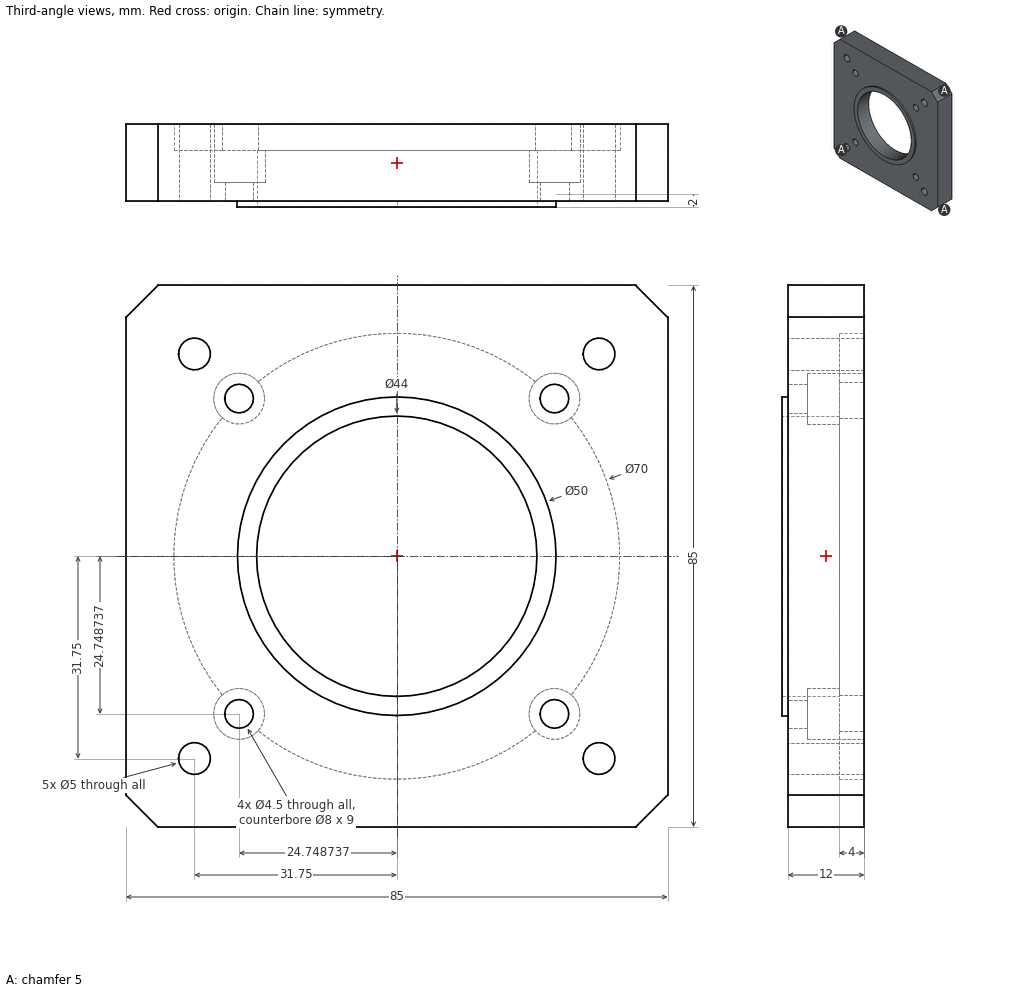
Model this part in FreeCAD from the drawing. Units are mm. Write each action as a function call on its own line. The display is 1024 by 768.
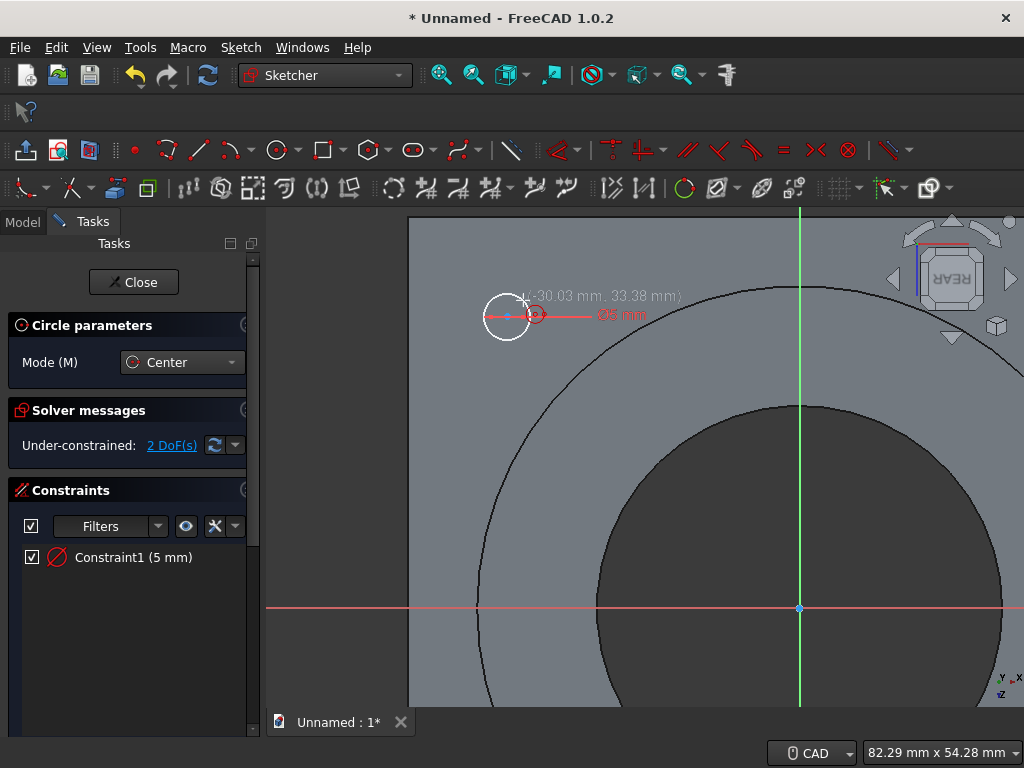
click(800, 608)
move(816, 592)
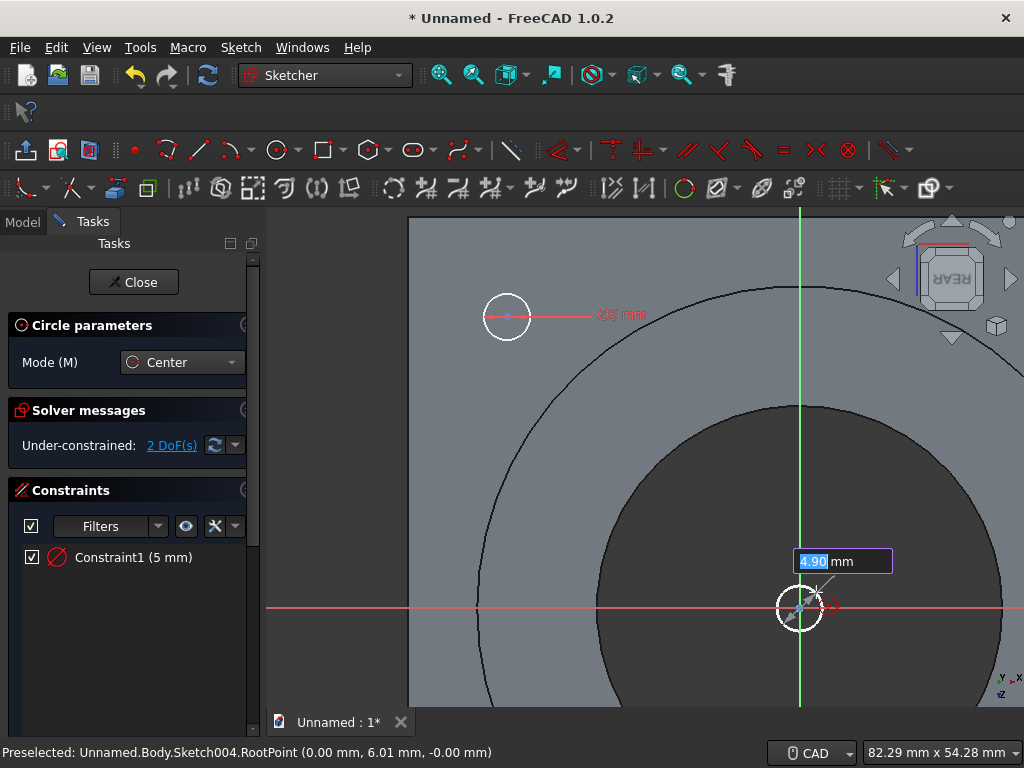
text(5)
key(Return)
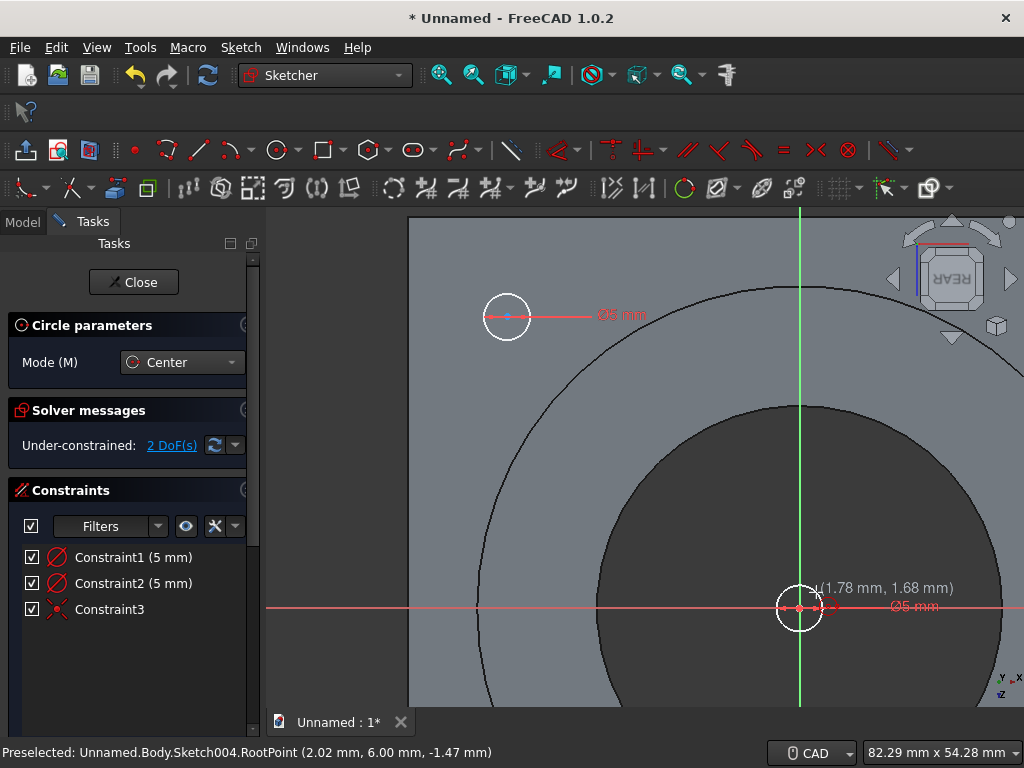
scroll(305, 273, down, 3)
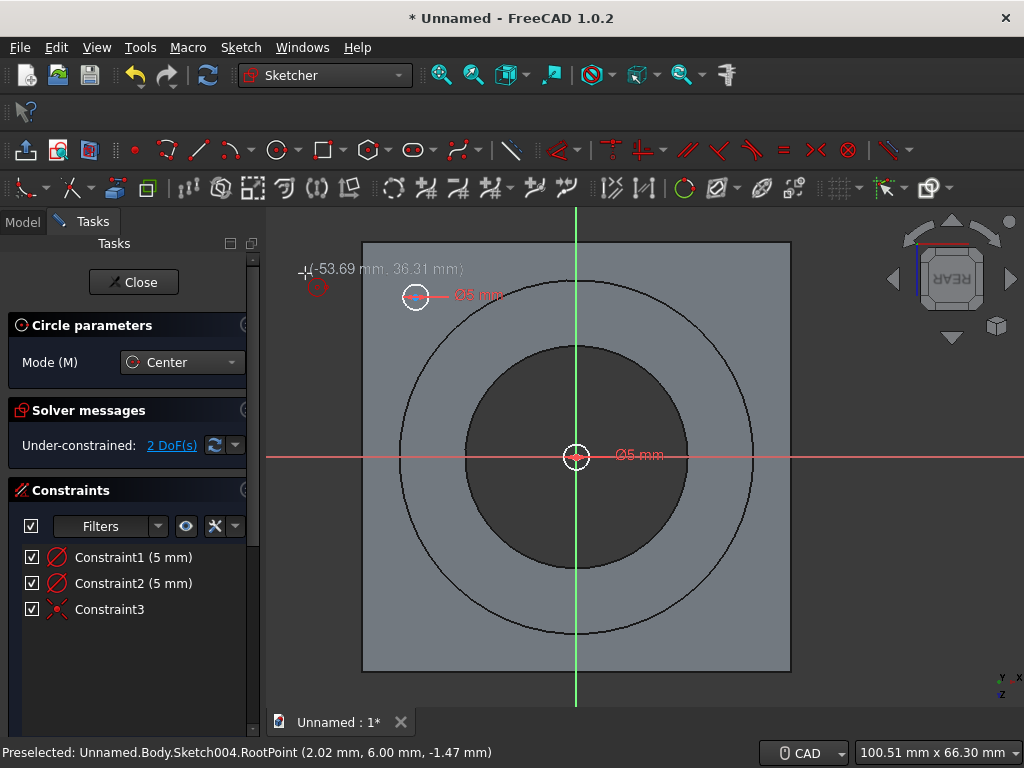
scroll(737, 618, up, 3)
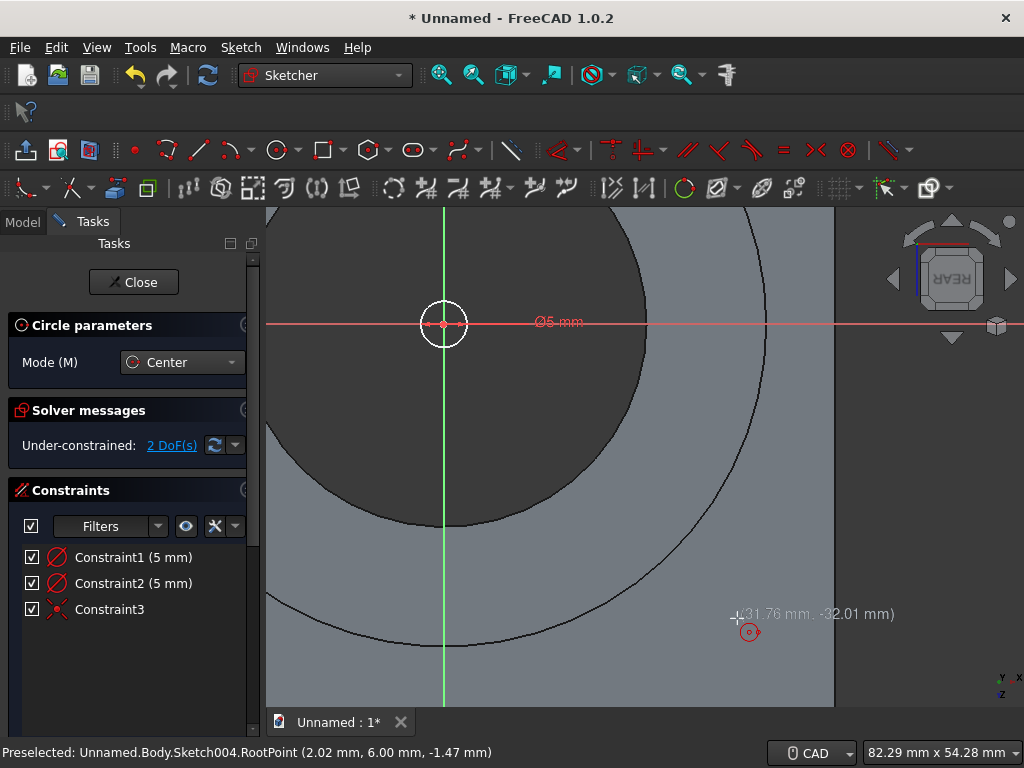
click(736, 617)
move(753, 600)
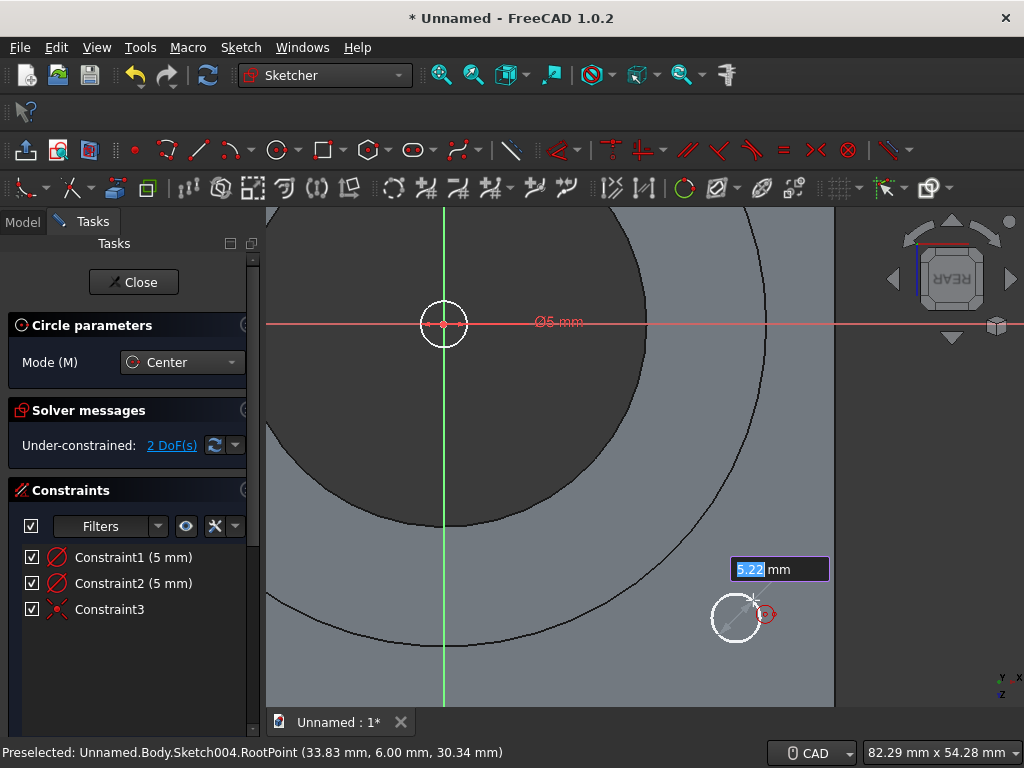
text(5)
key(Return)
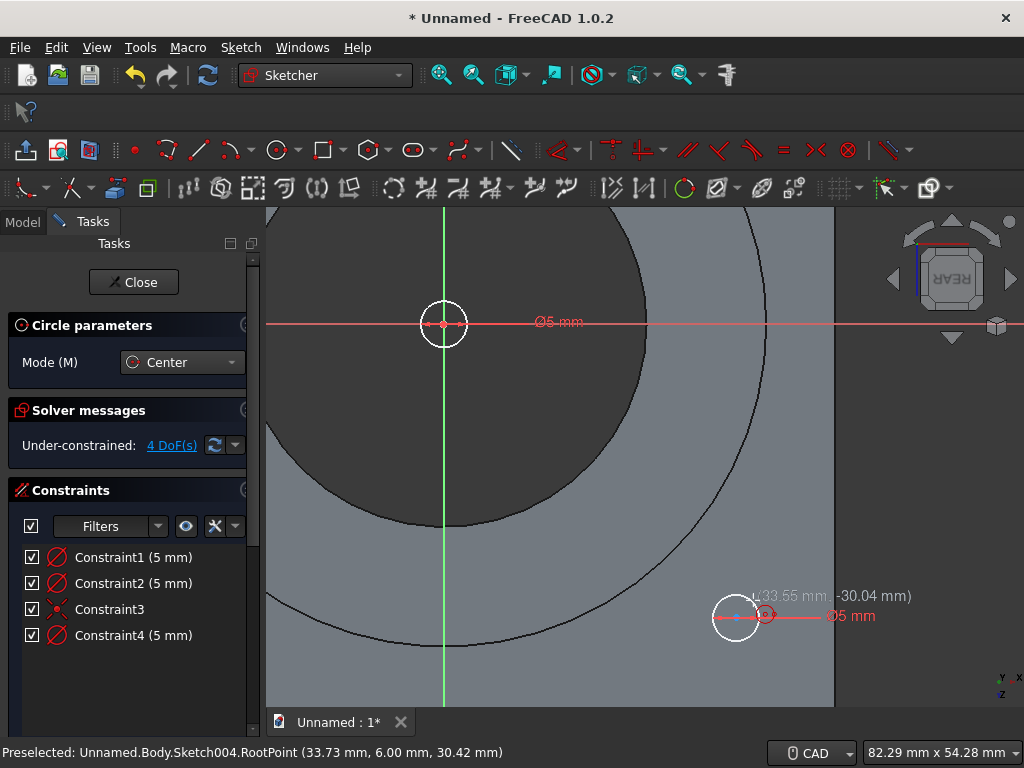
scroll(738, 618, down, 3)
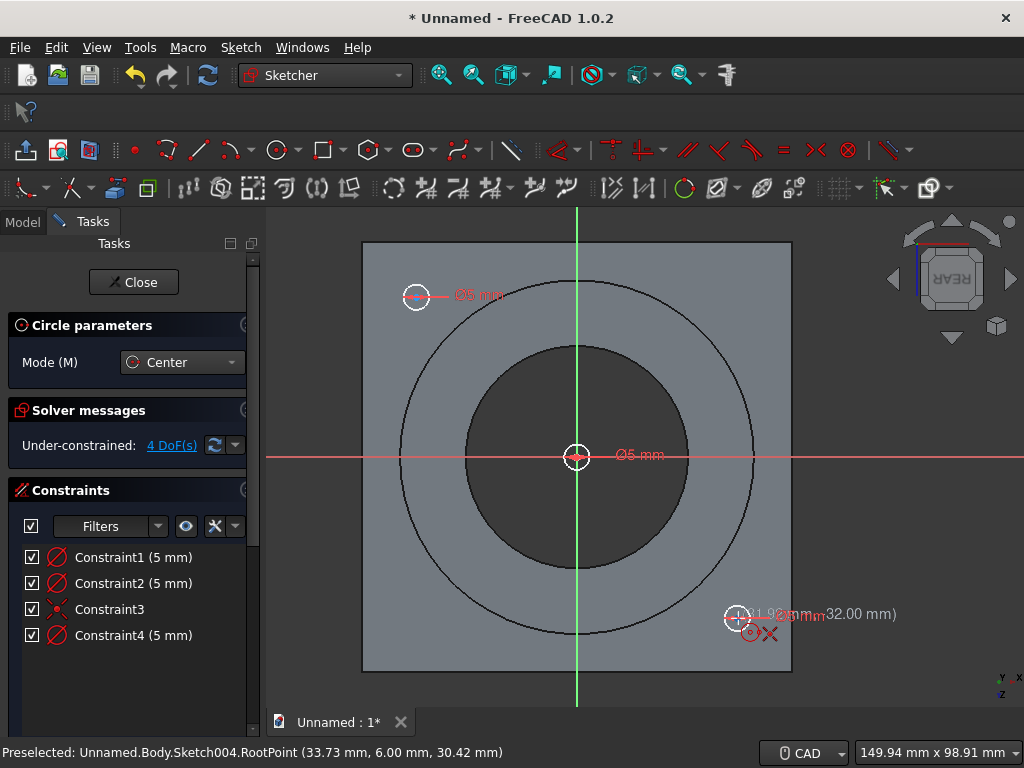
scroll(737, 297, up, 3)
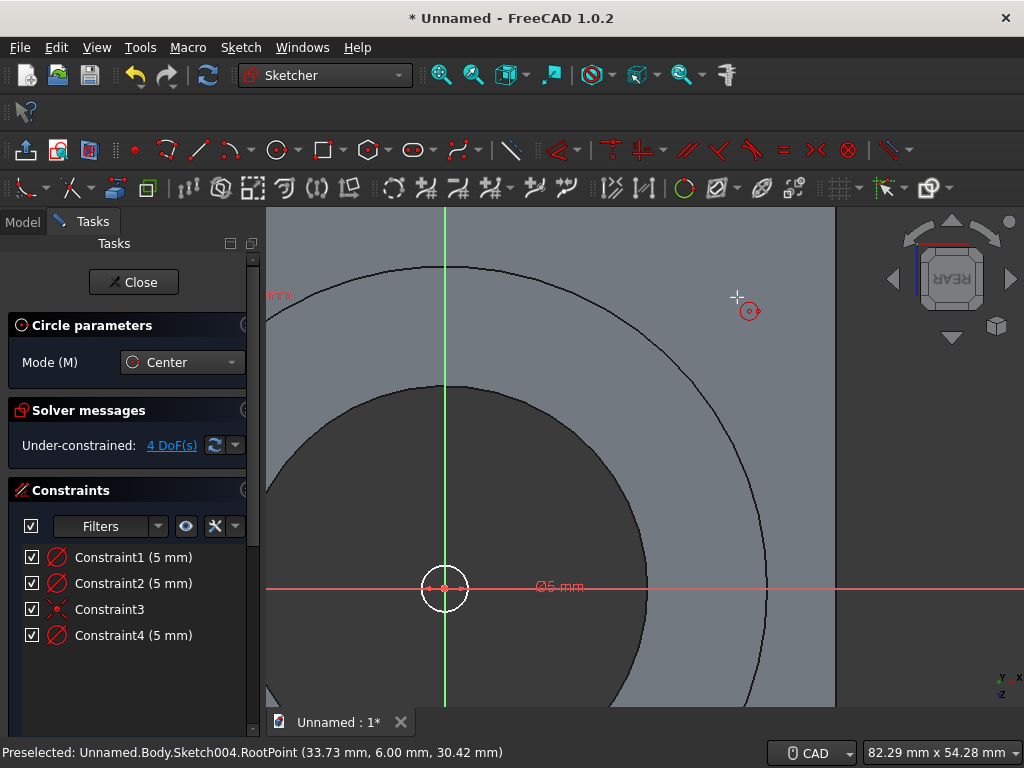
click(737, 296)
move(754, 280)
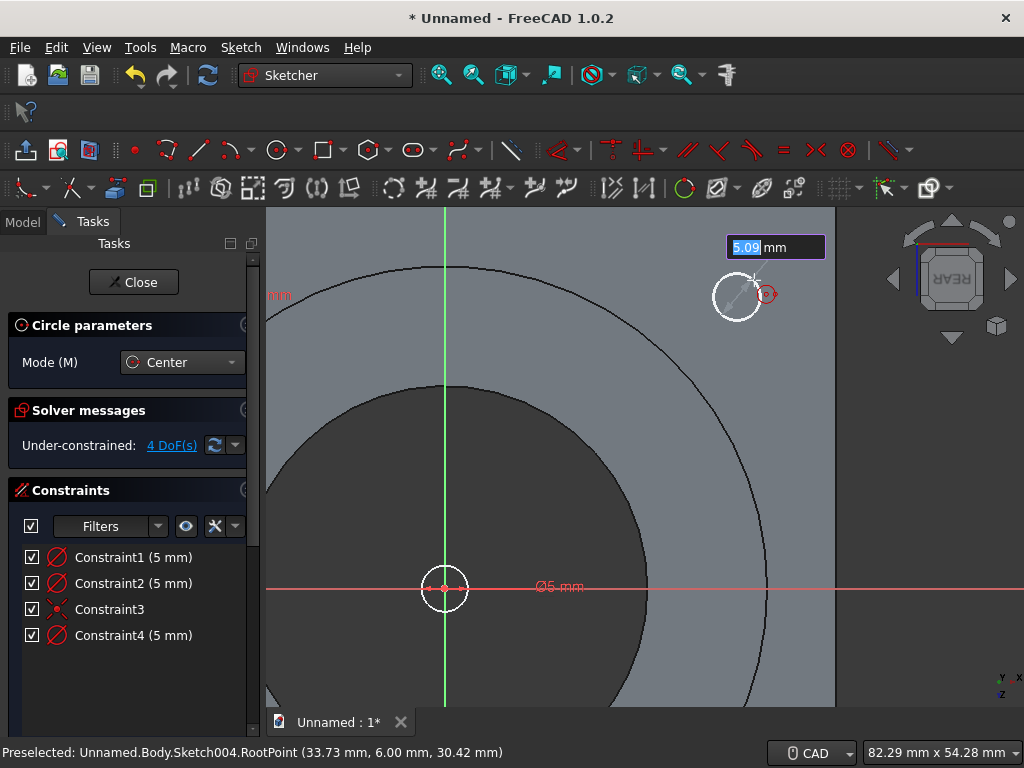
text(5)
key(Return)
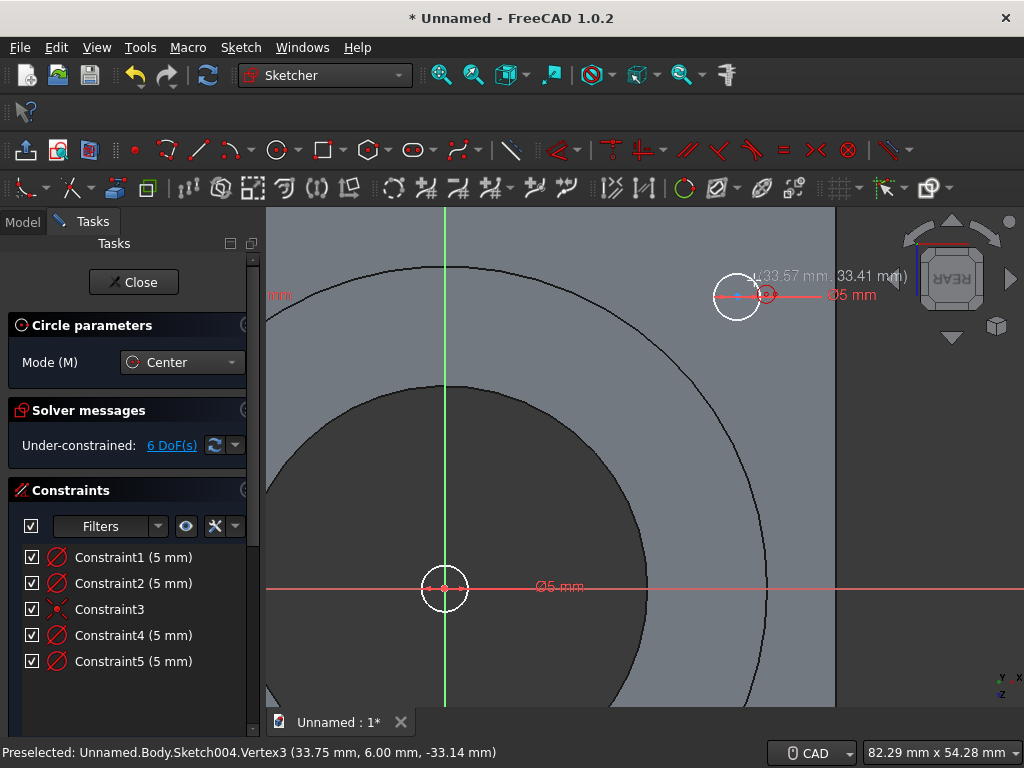
scroll(737, 297, down, 3)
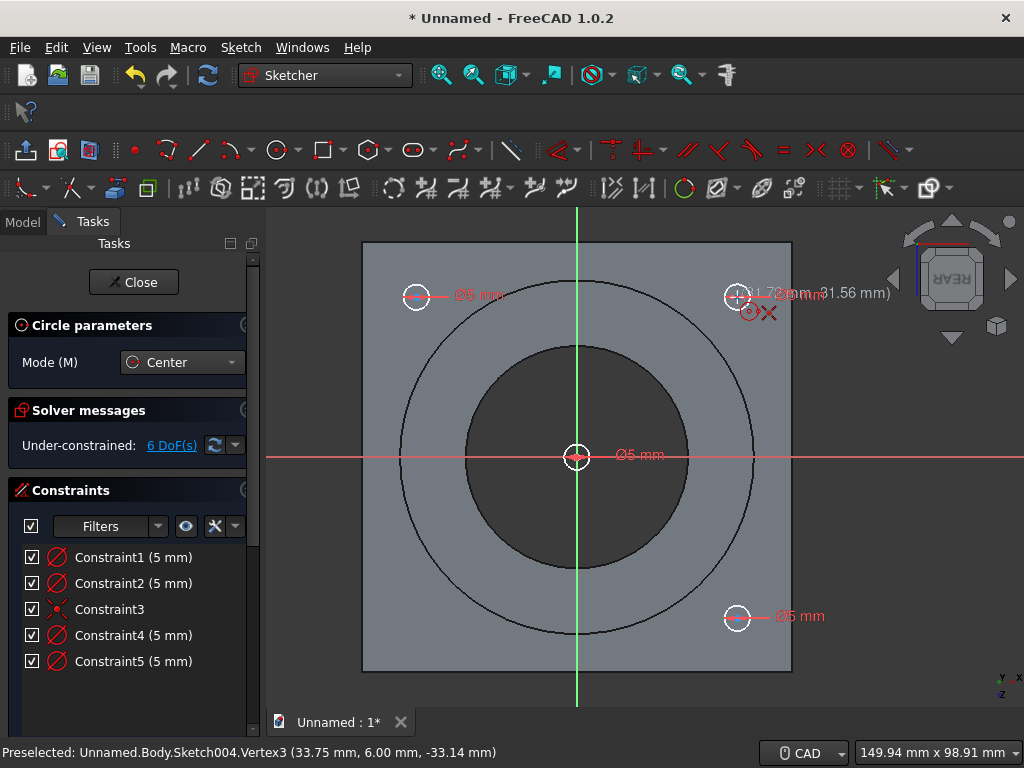
scroll(416, 618, up, 3)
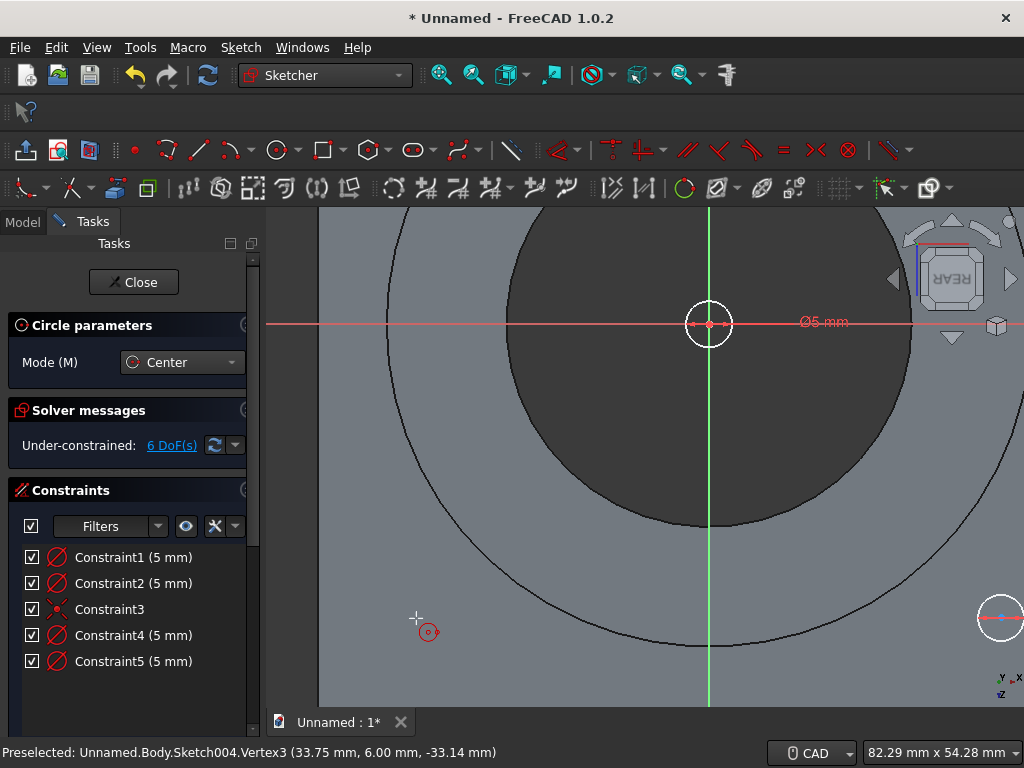
click(417, 617)
move(433, 600)